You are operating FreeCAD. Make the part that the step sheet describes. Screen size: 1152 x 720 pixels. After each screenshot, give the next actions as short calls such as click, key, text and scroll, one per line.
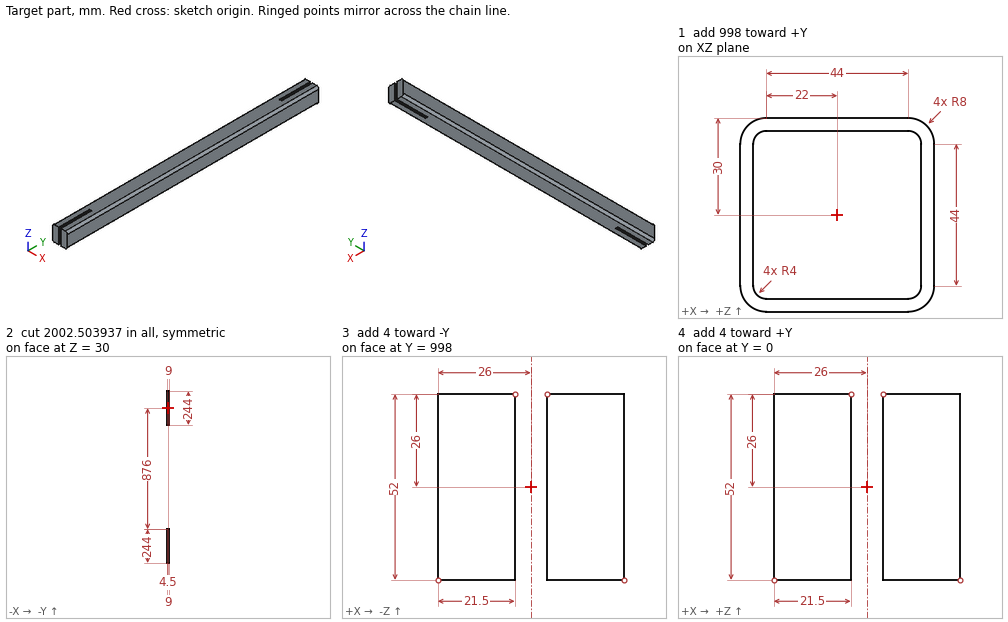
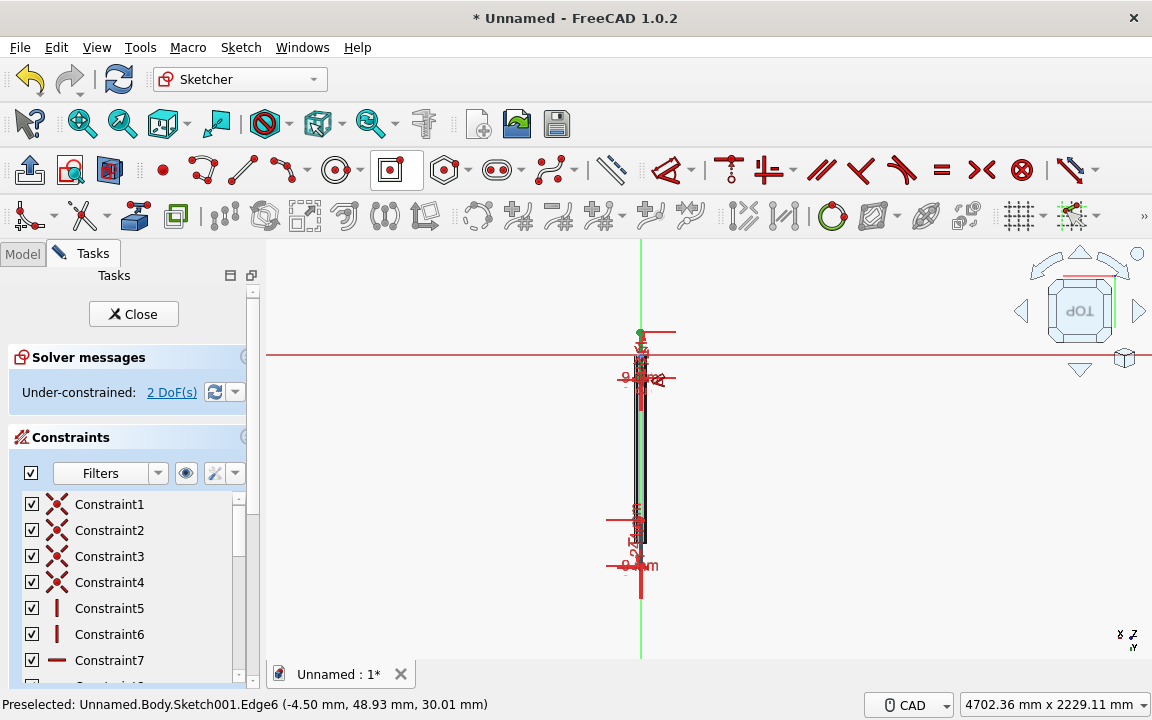
scroll(640, 520, up, 20)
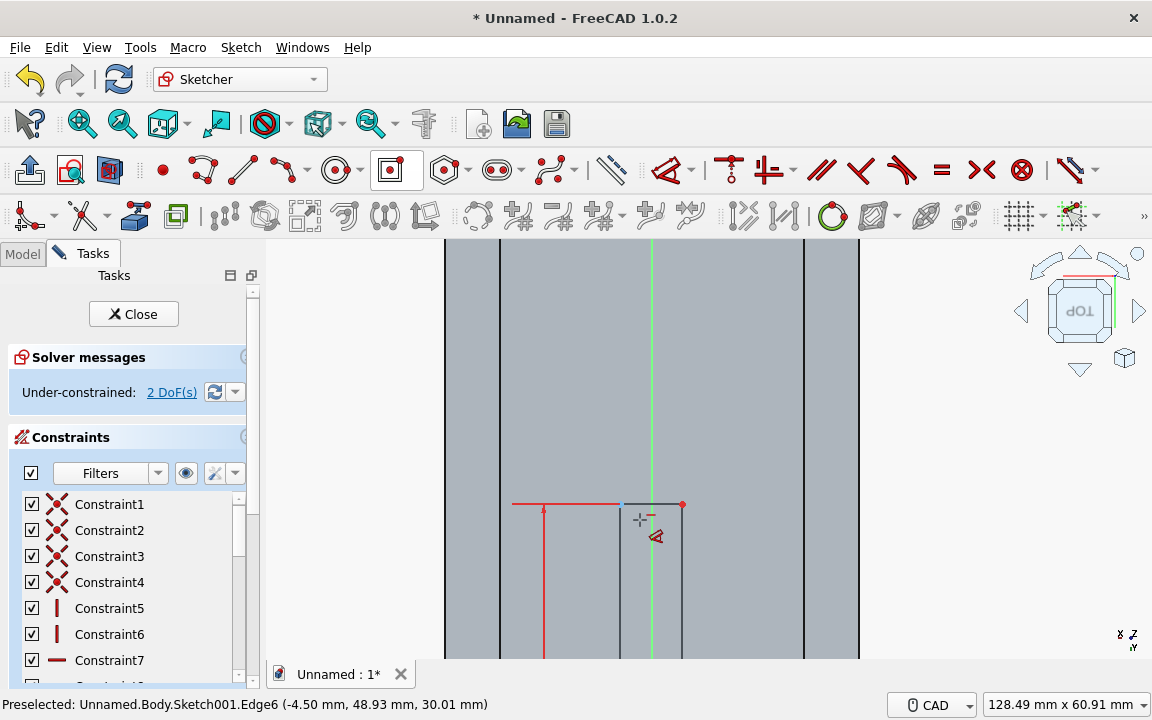
click(610, 496)
click(634, 530)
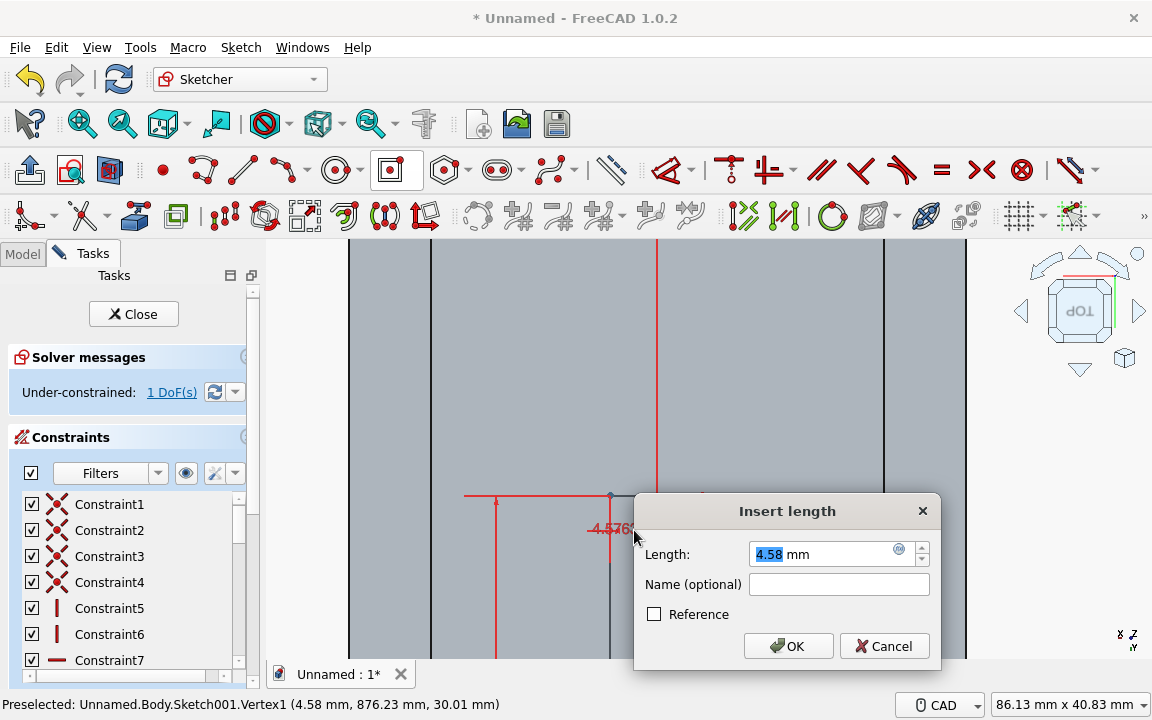
text(4.5)
key(Return)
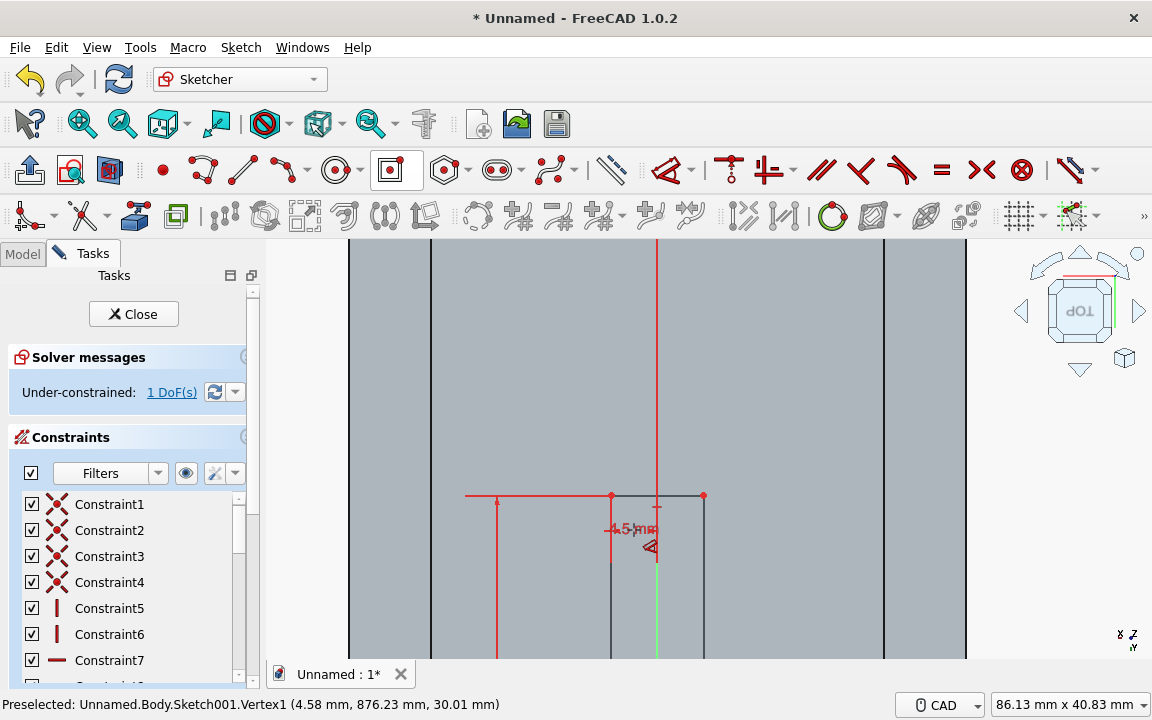
scroll(640, 449, down, 15)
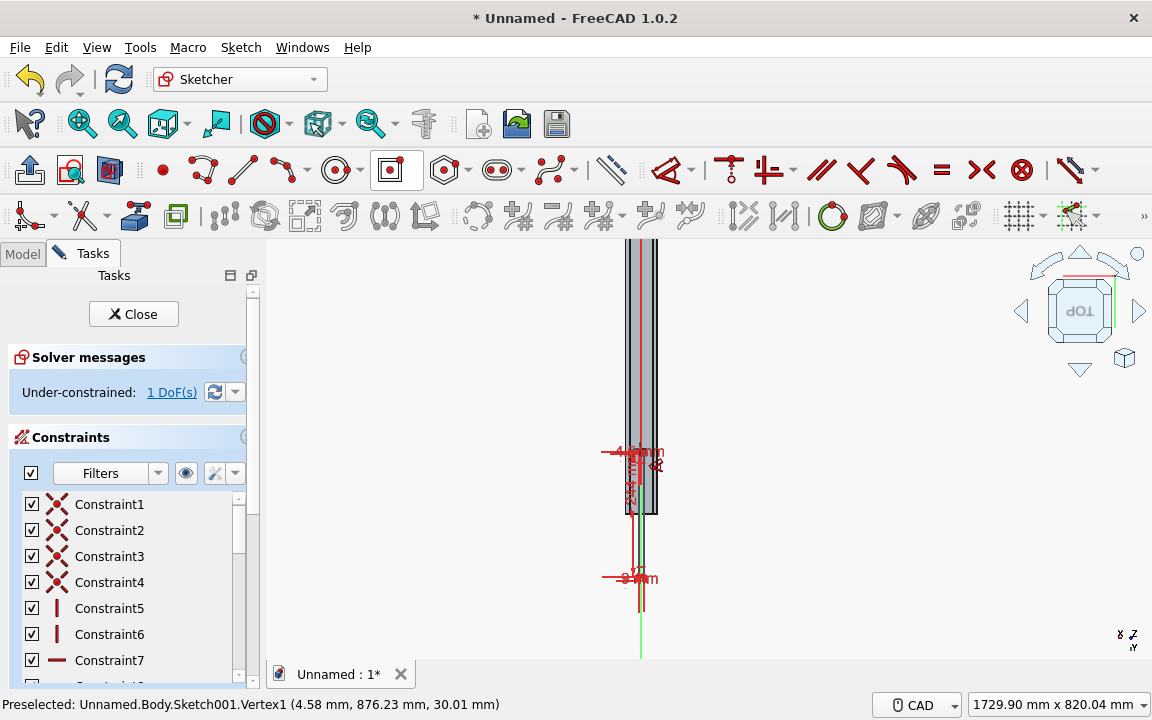
scroll(640, 560, down, 5)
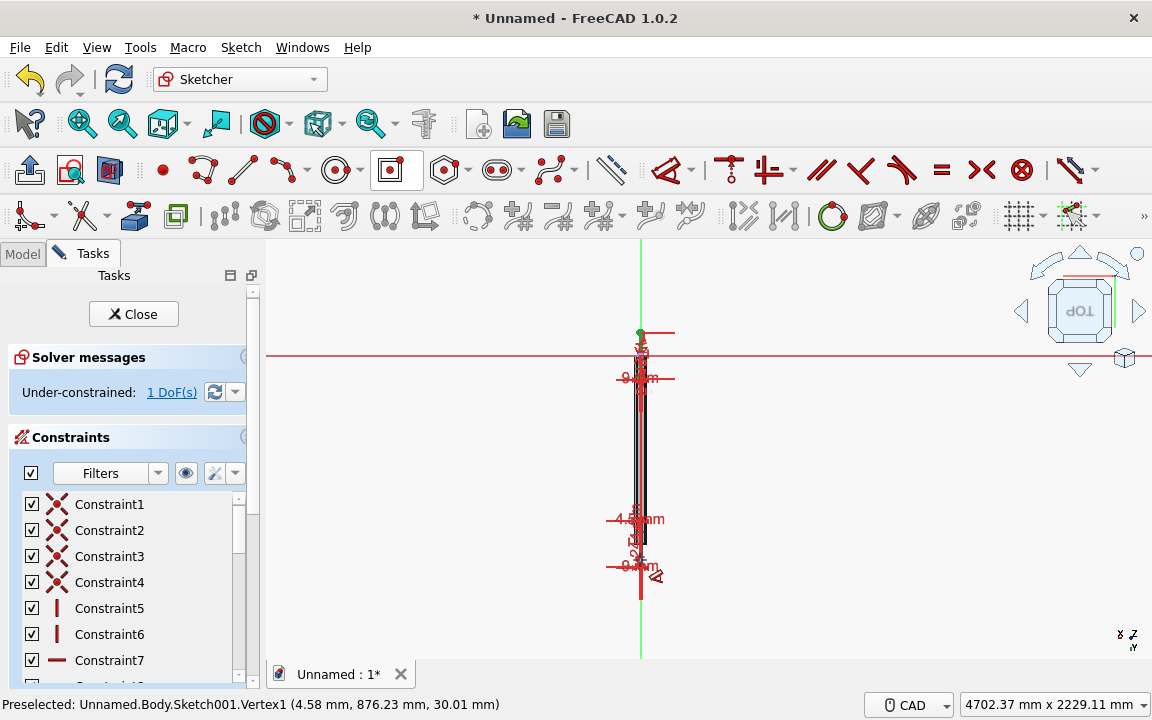
scroll(640, 521, up, 10)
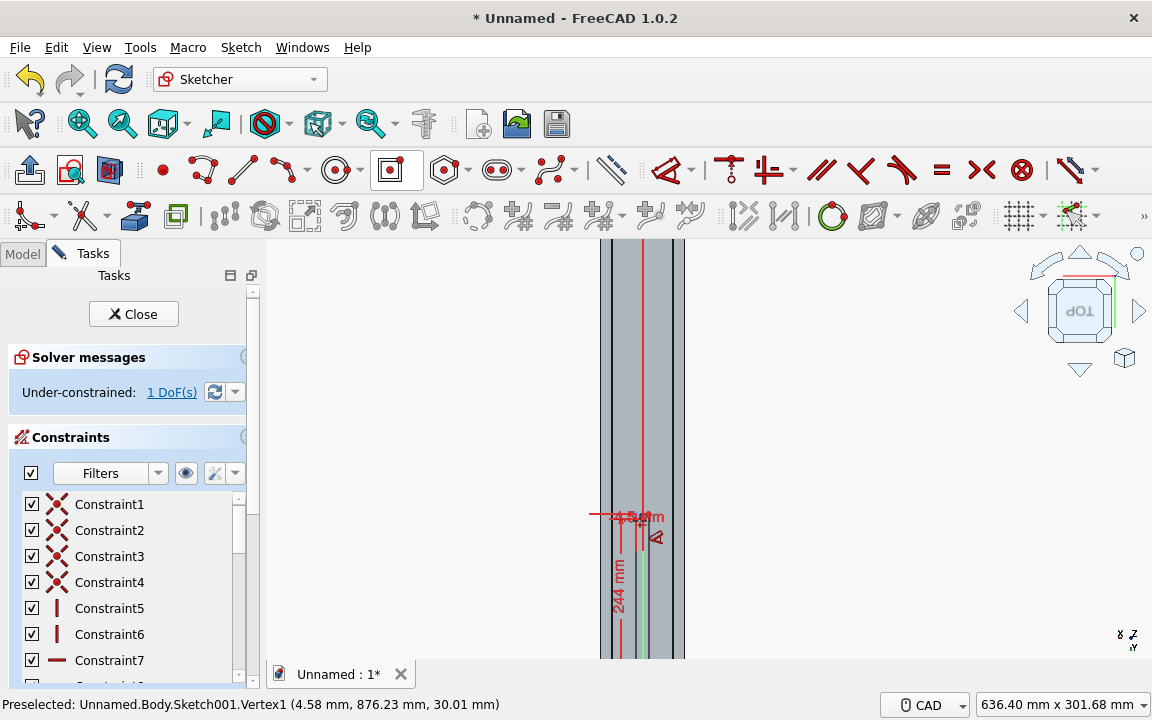
click(636, 514)
click(602, 391)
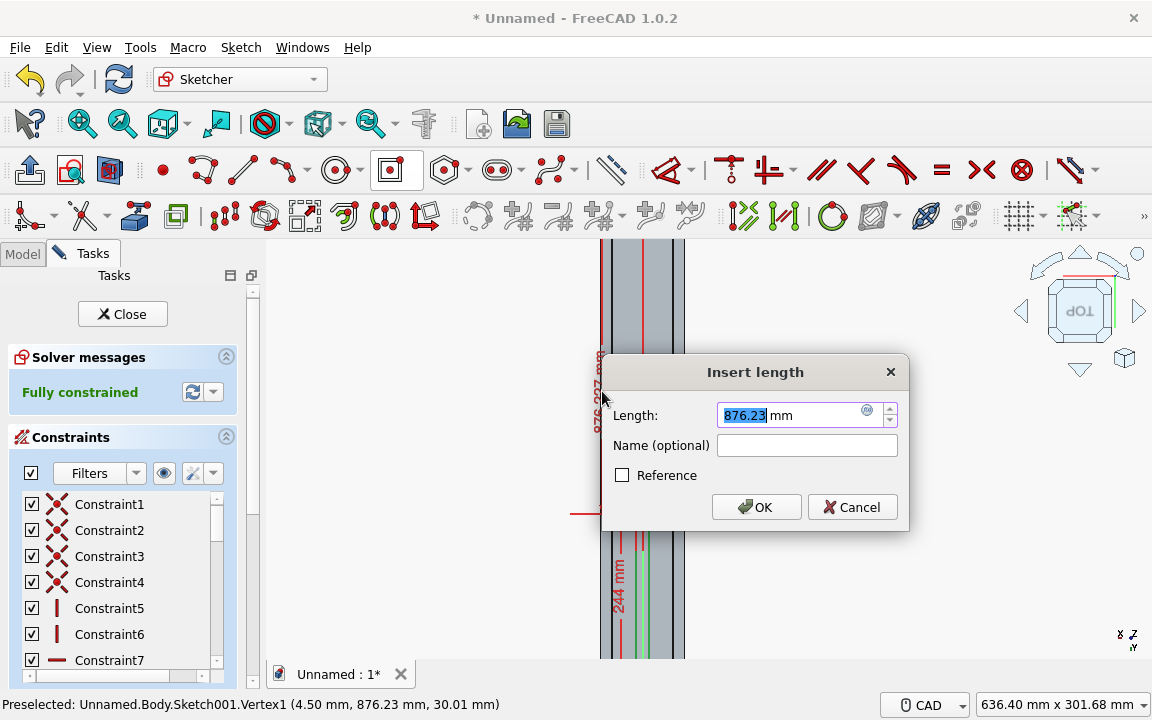
text(876)
key(Return)
key(Escape)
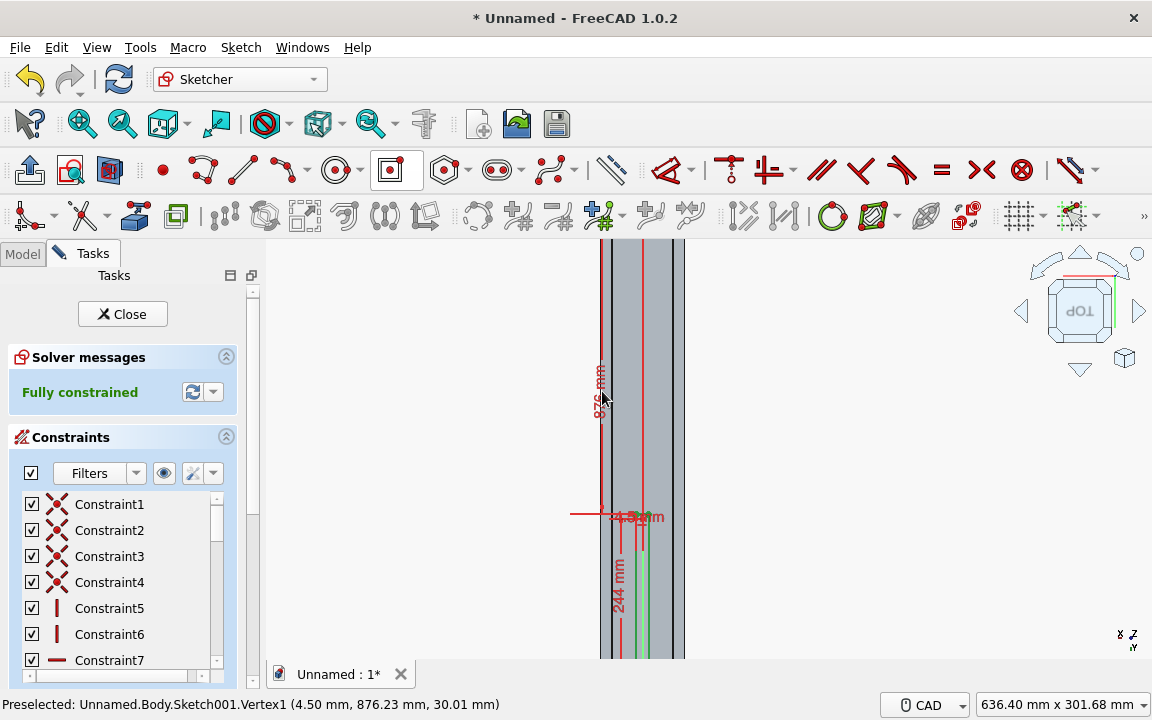
click(123, 314)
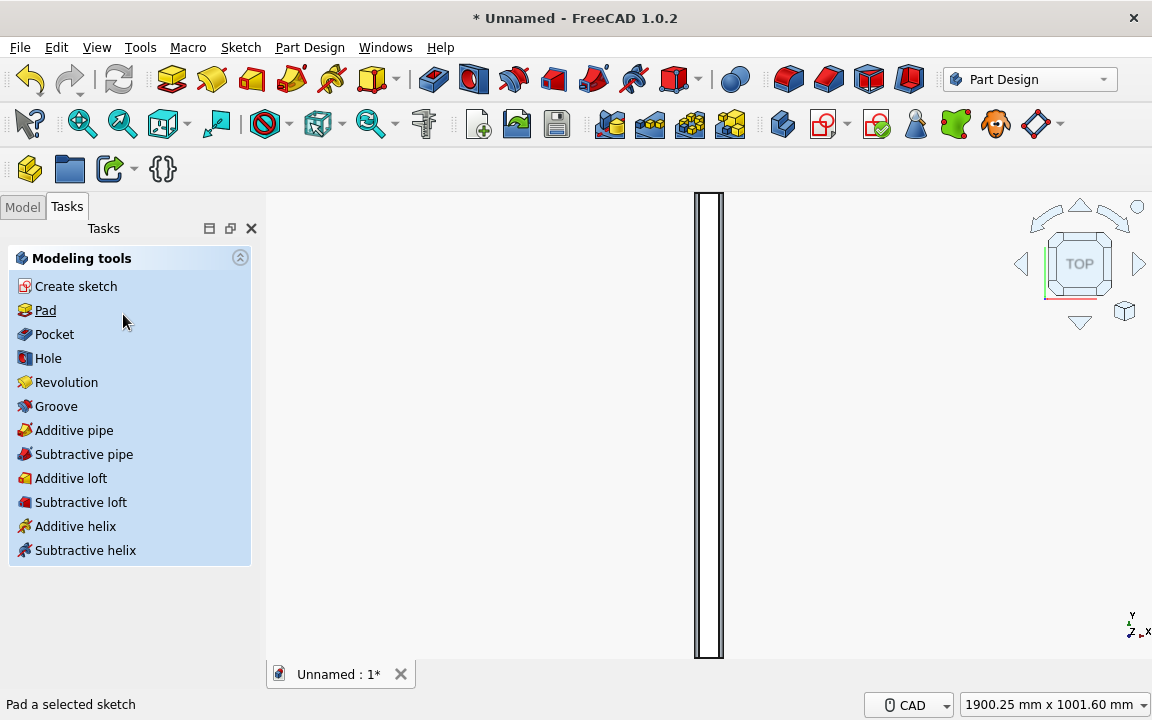
click(434, 80)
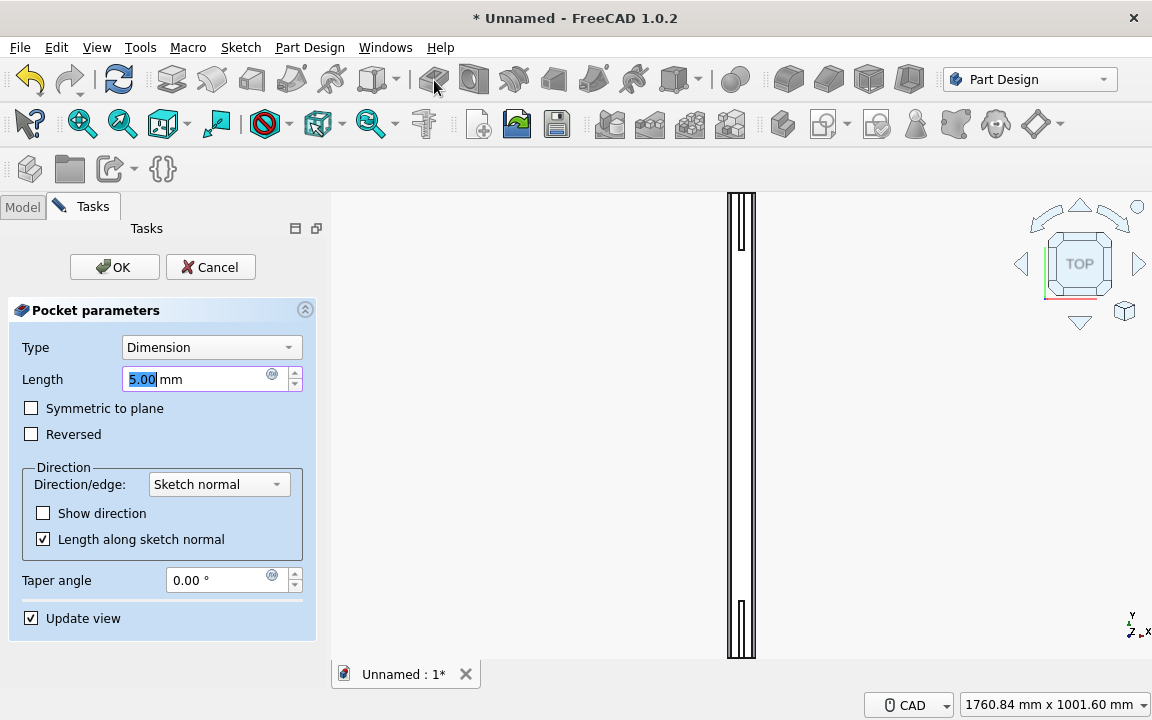
text(2002.503937)
key(Tab)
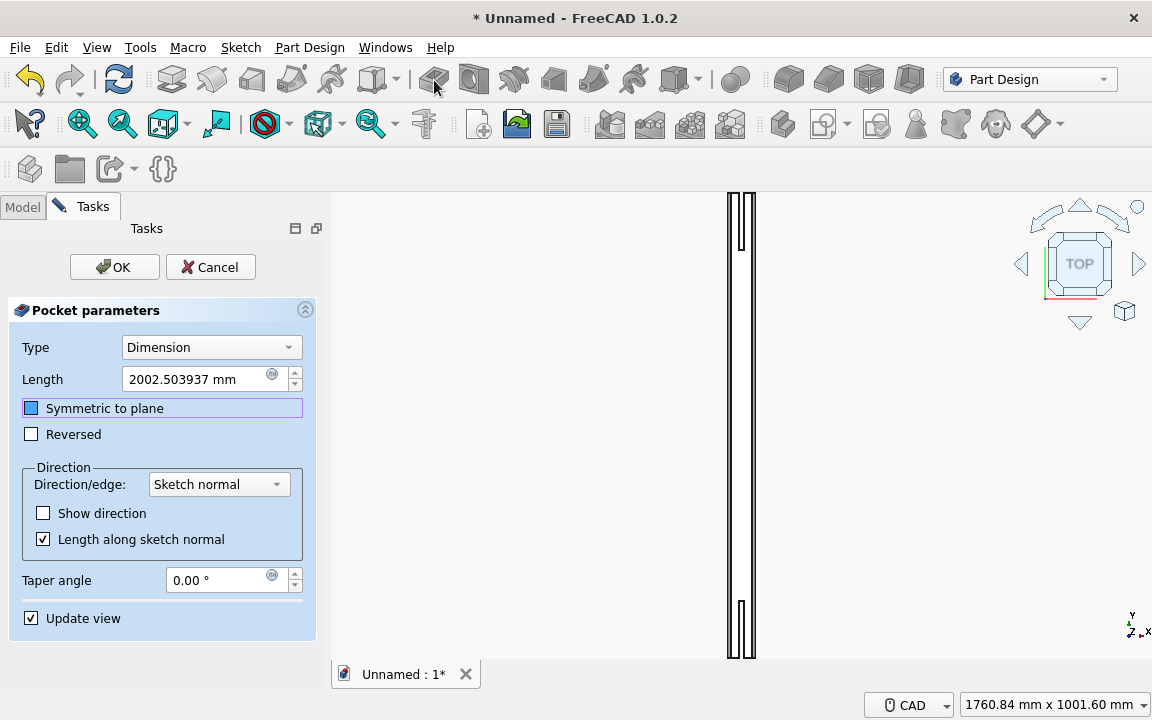
click(30, 408)